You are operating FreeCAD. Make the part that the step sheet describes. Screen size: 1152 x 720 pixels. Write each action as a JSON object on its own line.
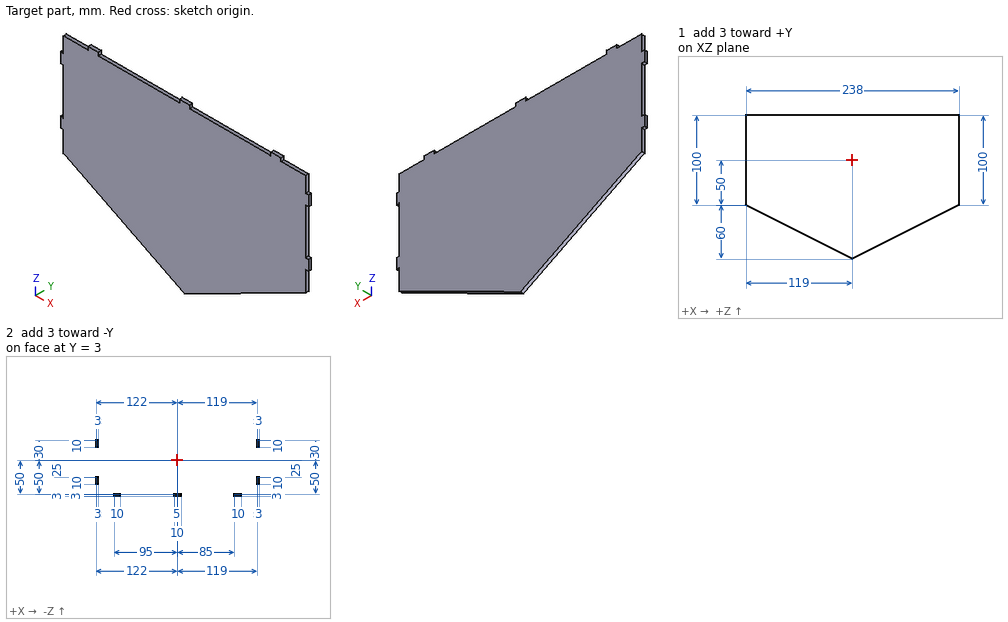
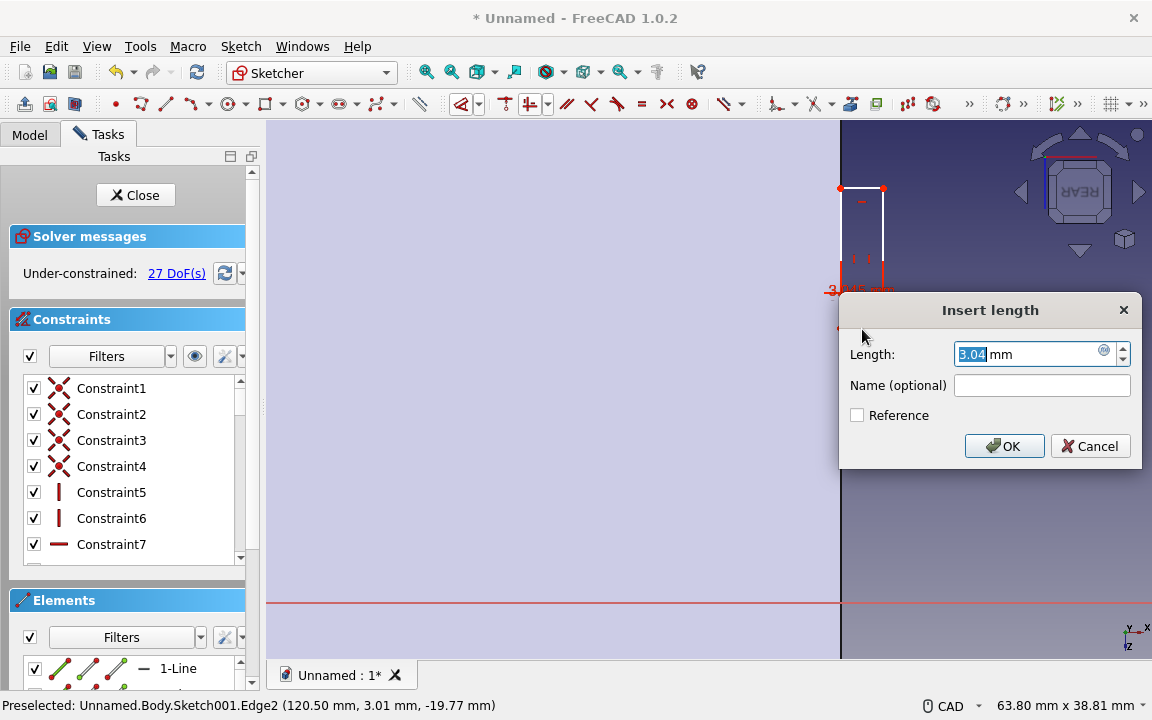
{"action": "type", "text": "3"}
{"action": "key", "text": "Return"}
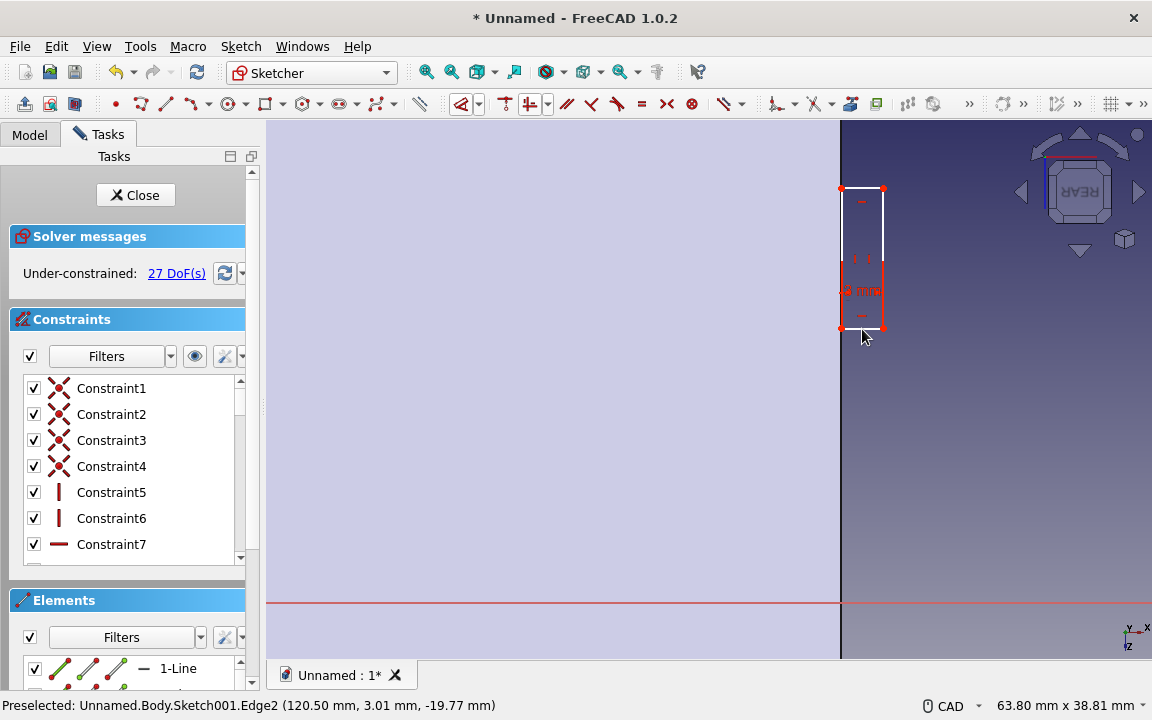
{"action": "scroll", "coordinate": [868, 331], "scroll_direction": "down", "scroll_amount": 10}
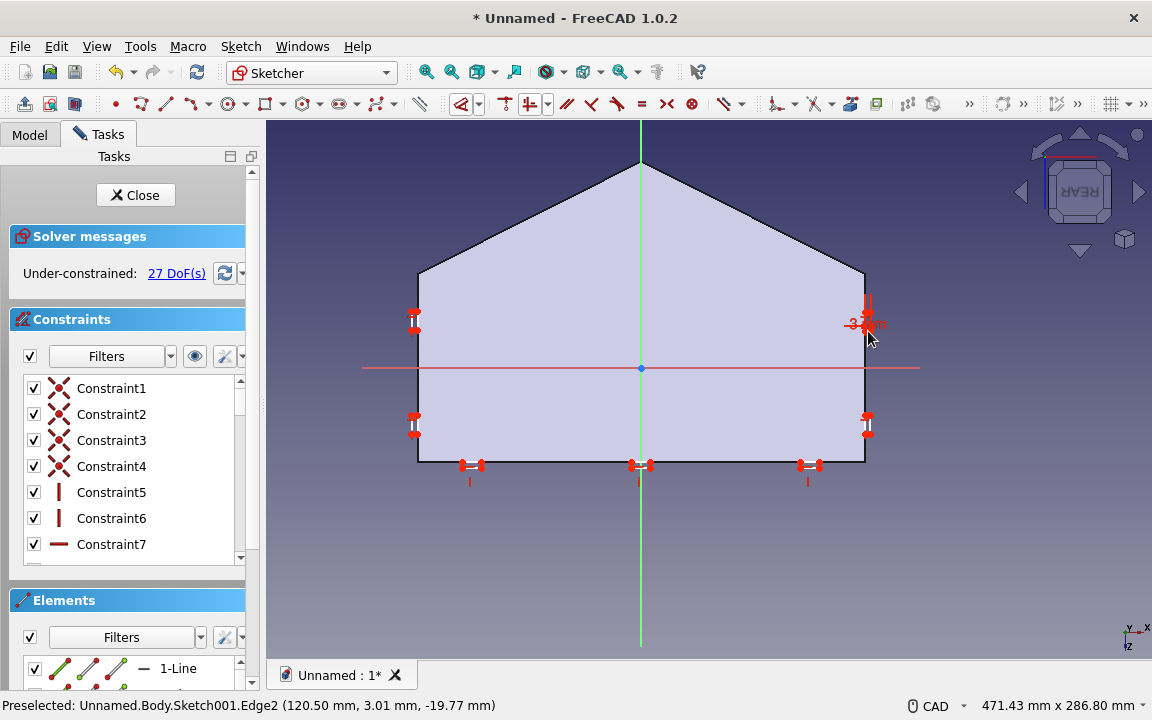
{"action": "scroll", "coordinate": [867, 434], "scroll_direction": "up", "scroll_amount": 11}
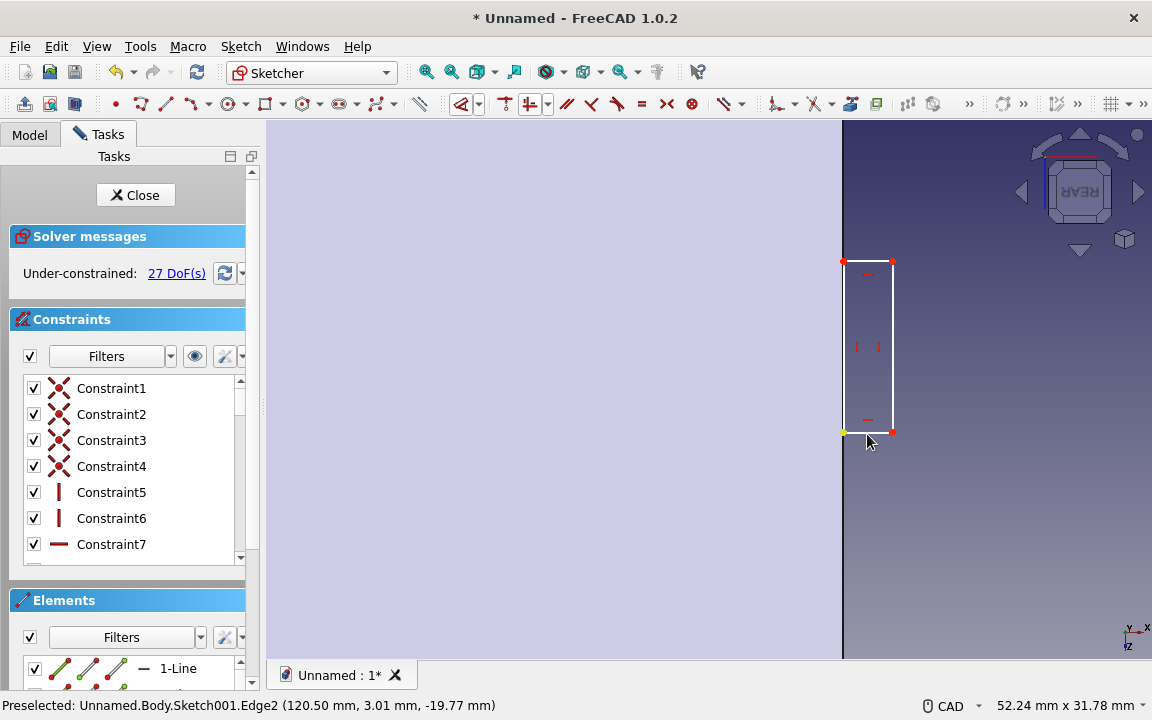
{"action": "left_click", "coordinate": [859, 433]}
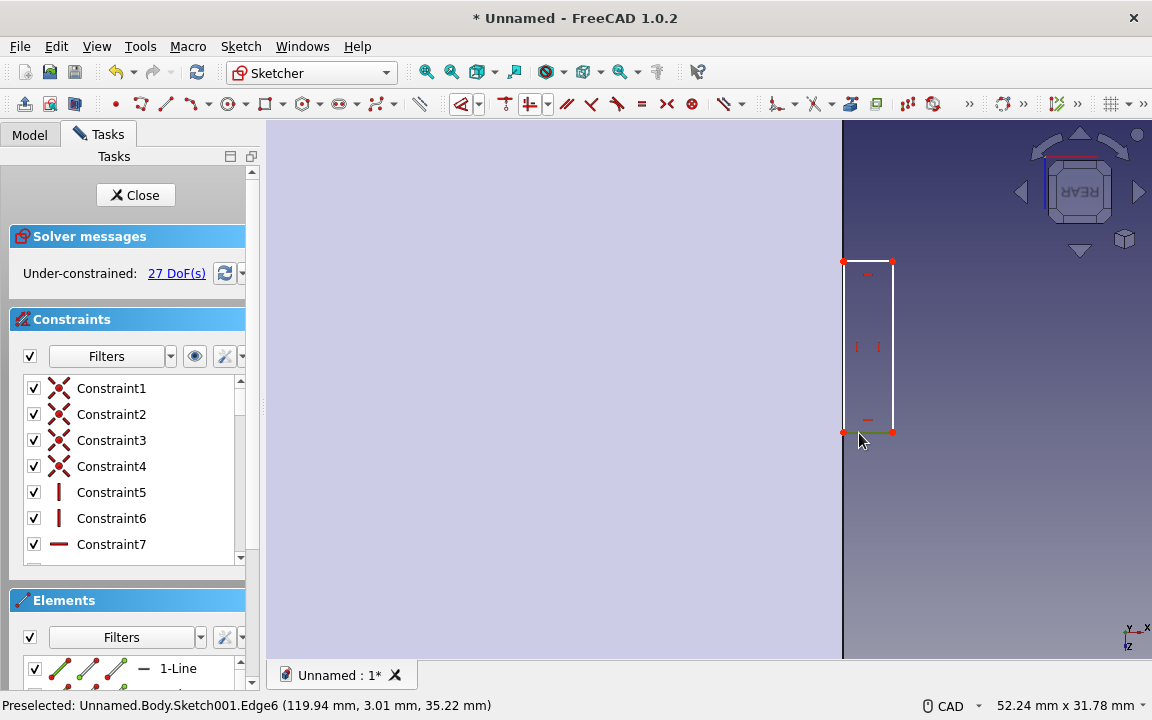
{"action": "key", "text": "l"}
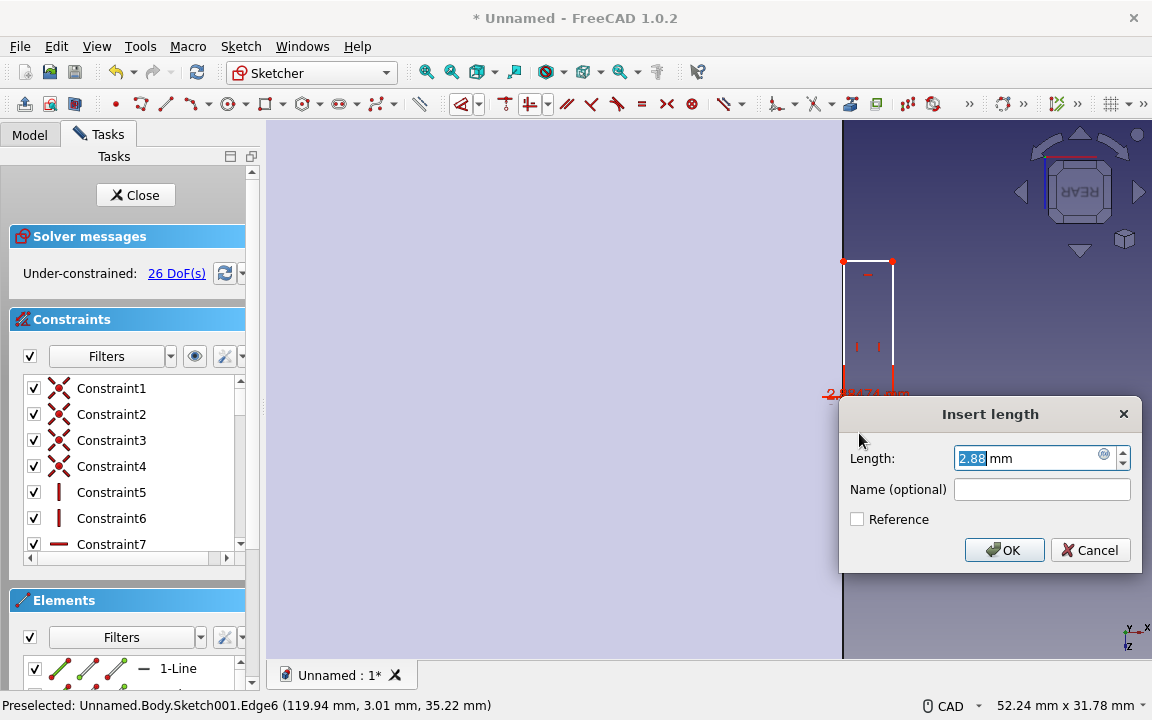
{"action": "type", "text": "3"}
{"action": "key", "text": "Return"}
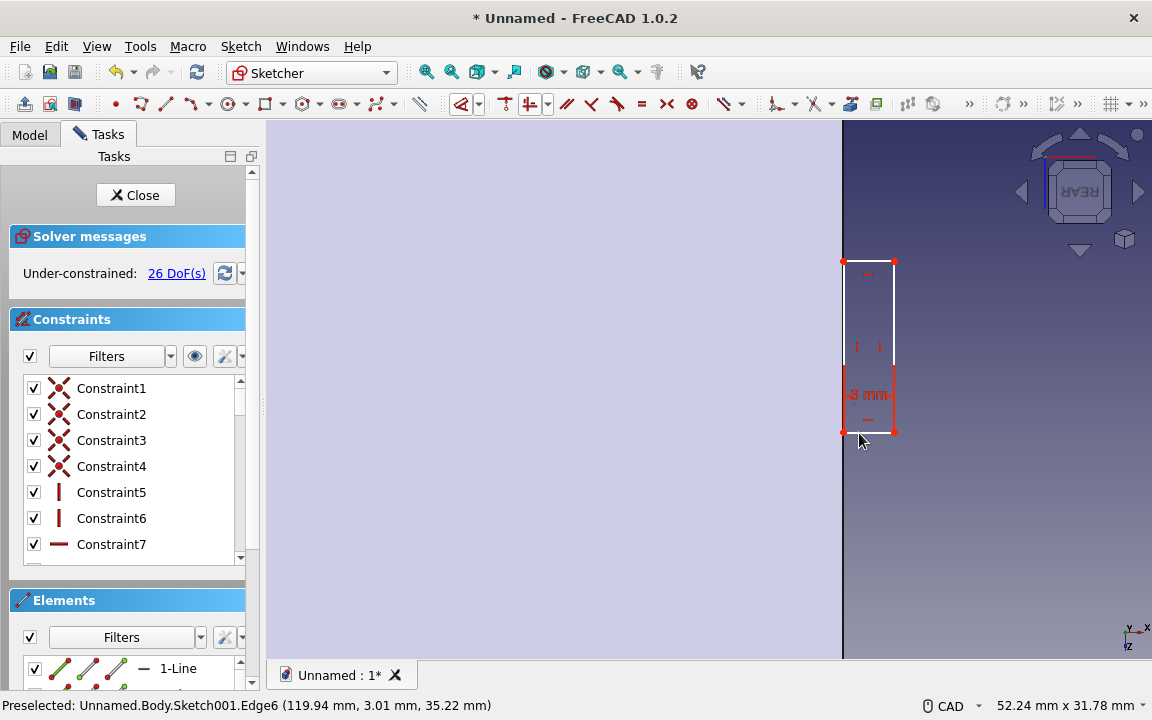
{"action": "scroll", "coordinate": [867, 434], "scroll_direction": "down", "scroll_amount": 11}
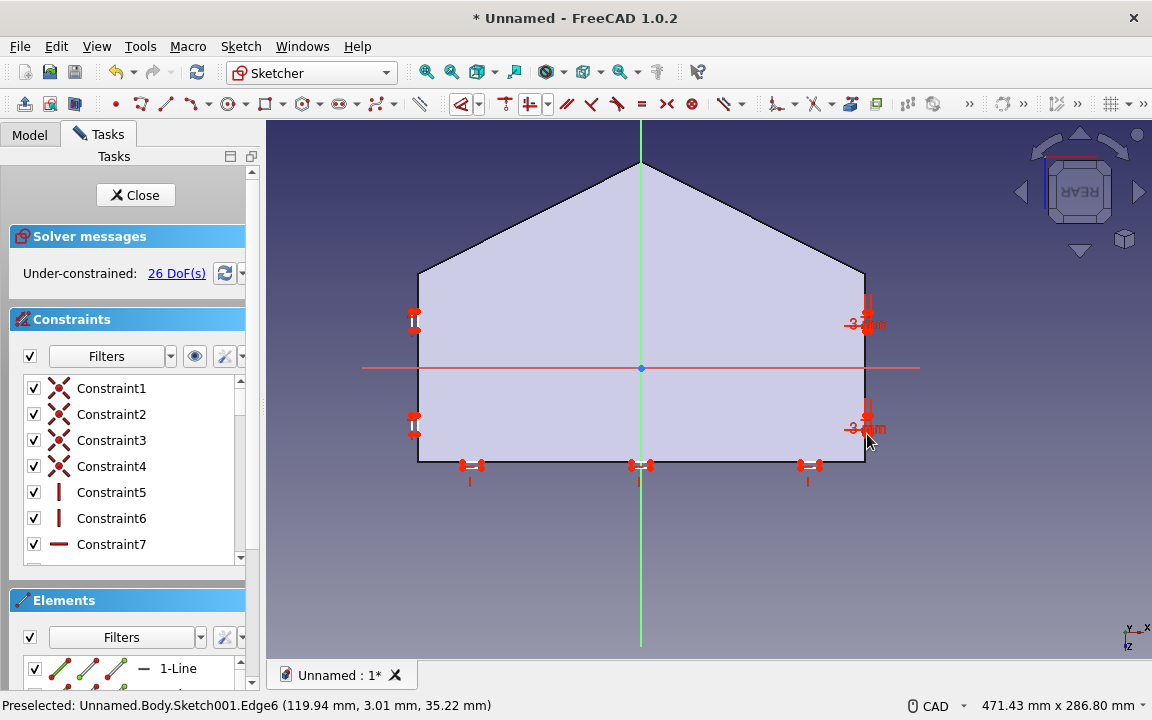
{"action": "scroll", "coordinate": [414, 434], "scroll_direction": "up", "scroll_amount": 11}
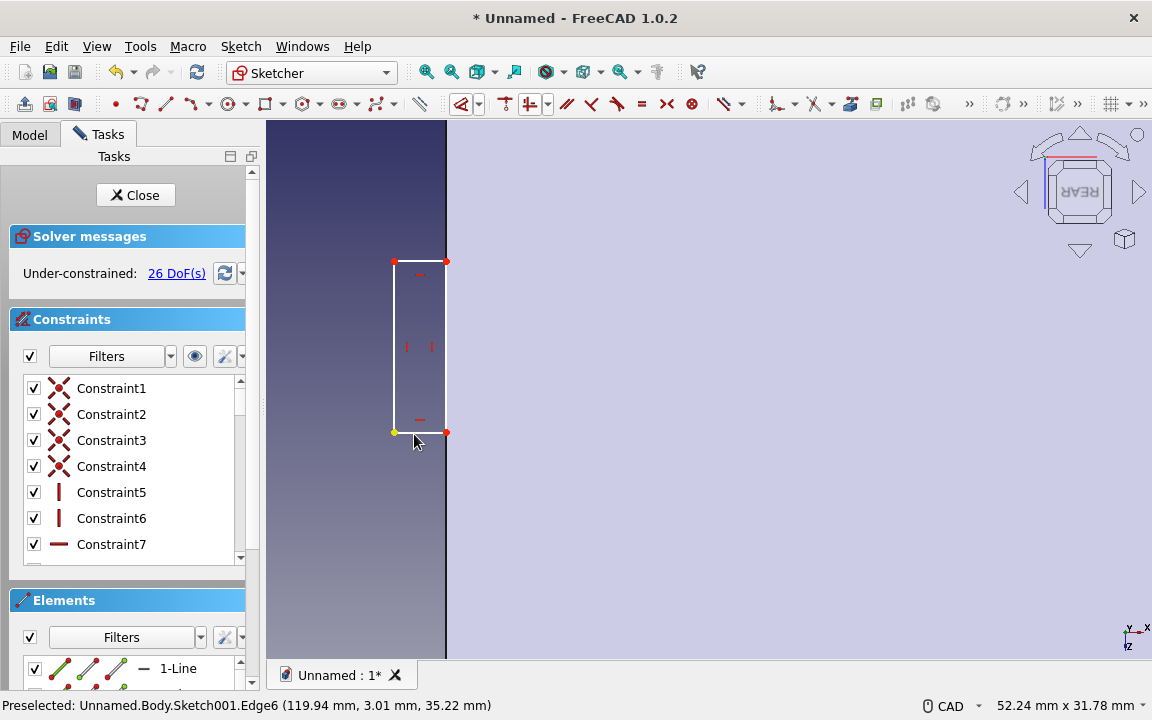
{"action": "left_click", "coordinate": [410, 433]}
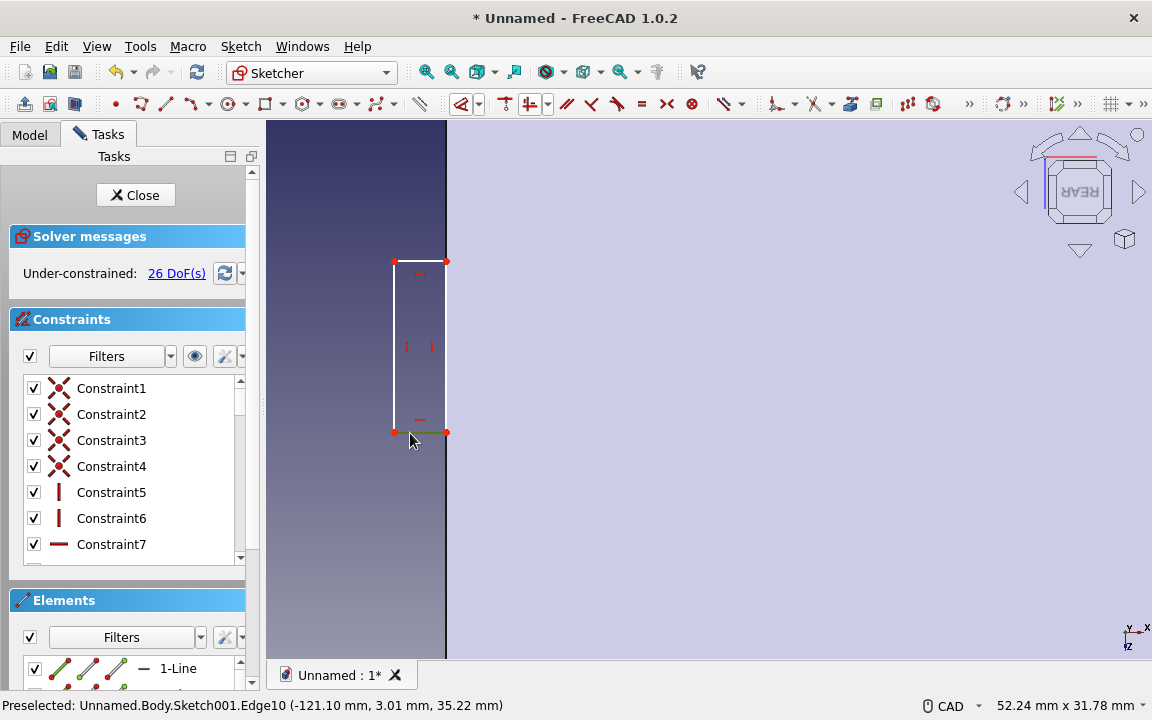
{"action": "key", "text": "l"}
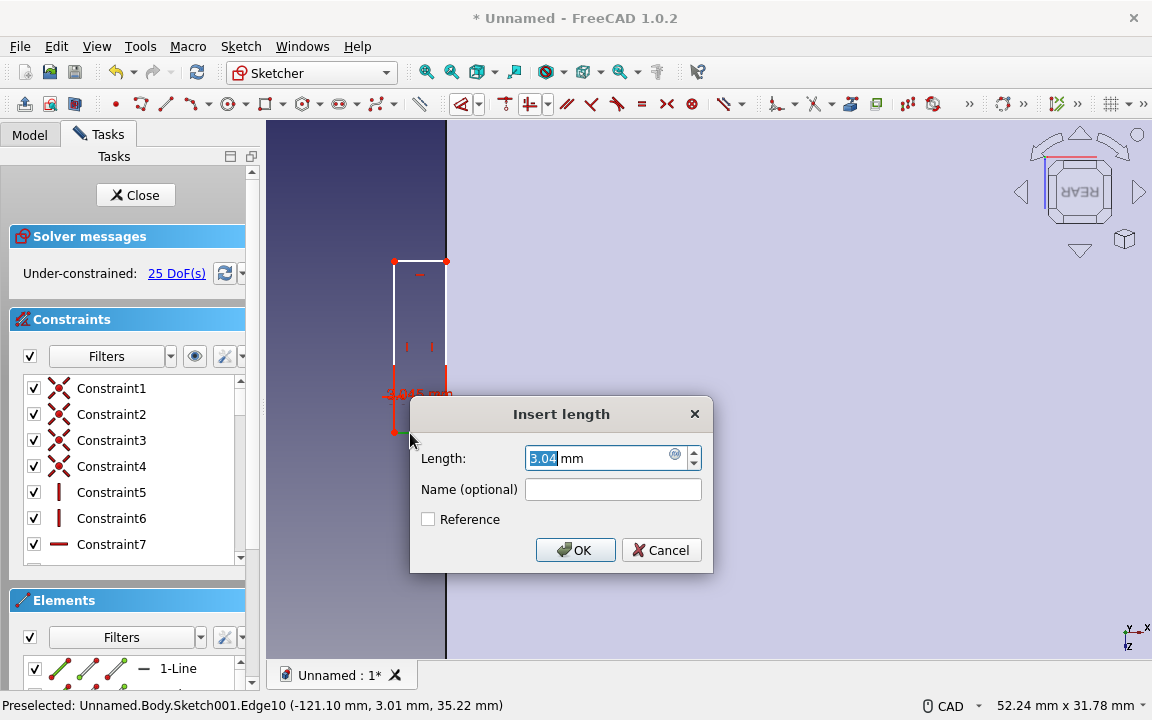
{"action": "type", "text": "3"}
{"action": "key", "text": "Return"}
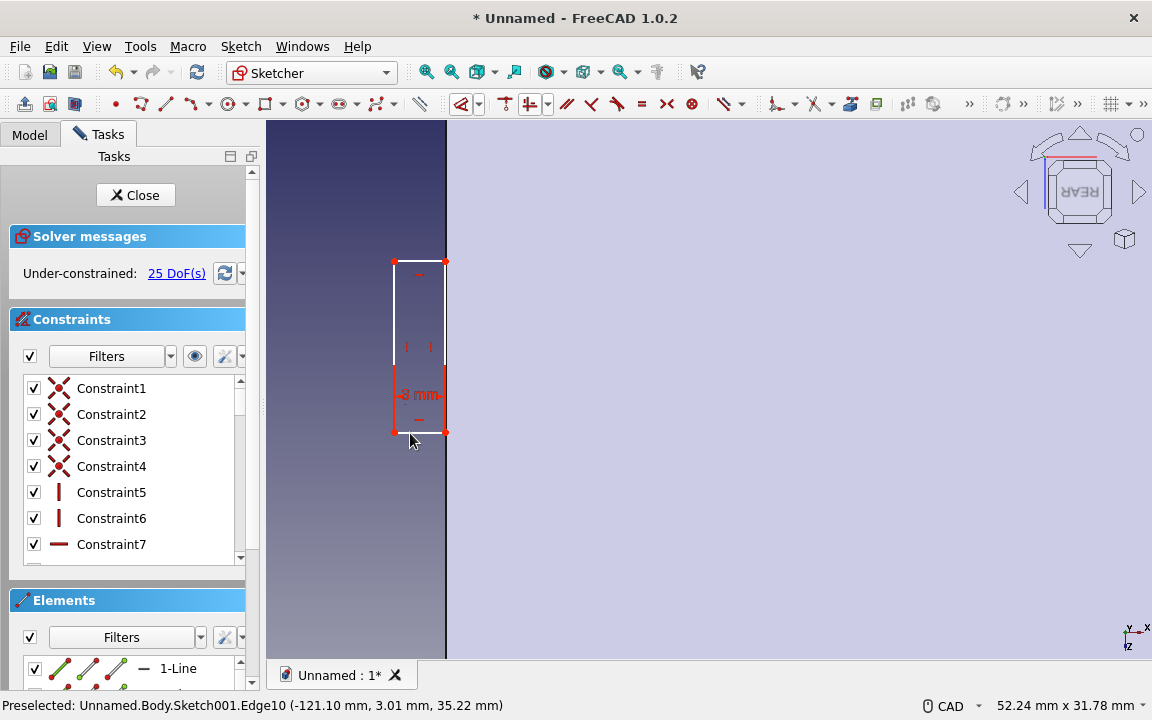
{"action": "scroll", "coordinate": [413, 434], "scroll_direction": "down", "scroll_amount": 11}